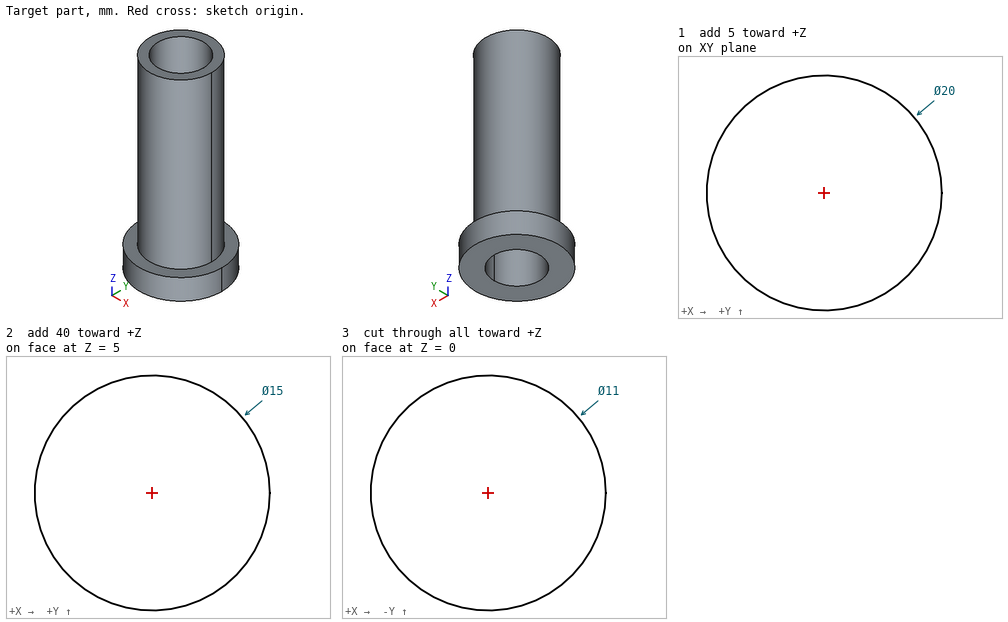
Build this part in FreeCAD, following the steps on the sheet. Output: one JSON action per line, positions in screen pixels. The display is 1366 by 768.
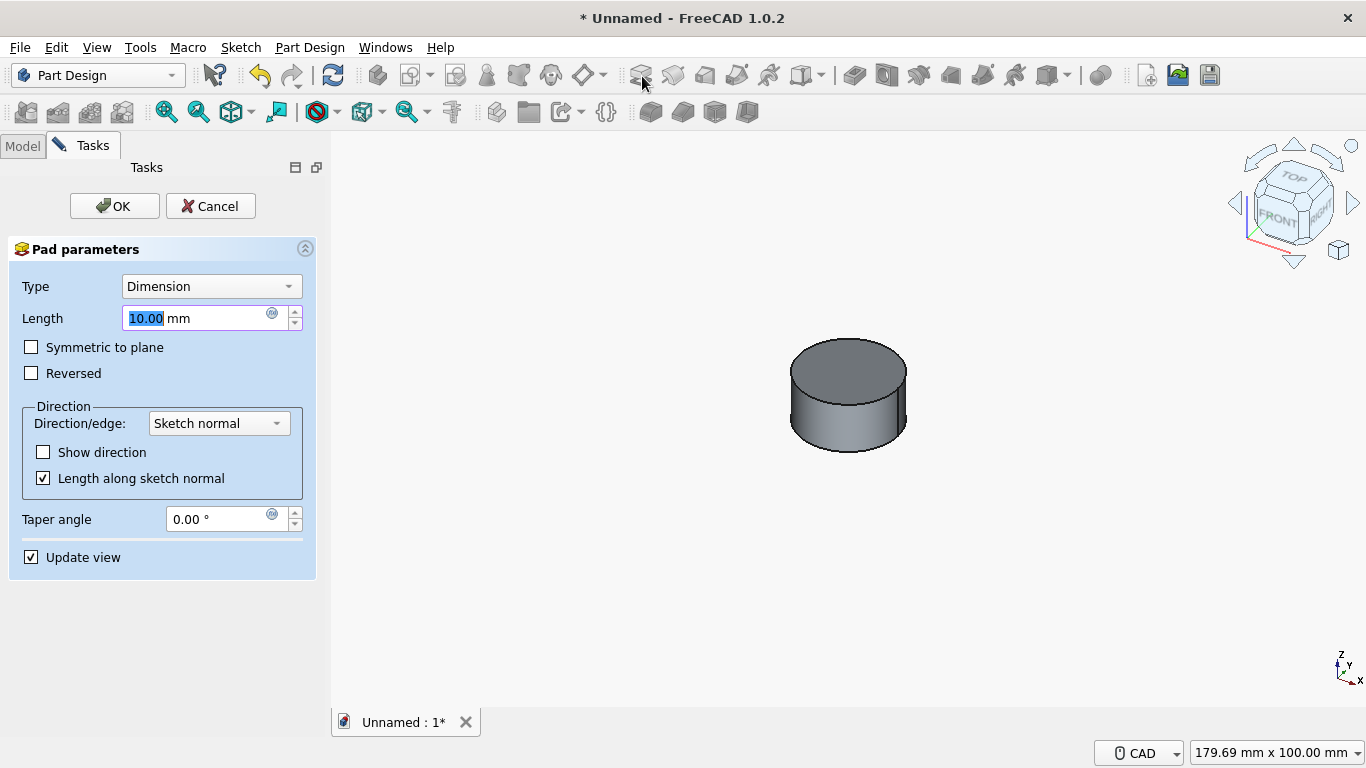
{"action": "type", "text": "5"}
{"action": "key", "text": "Tab"}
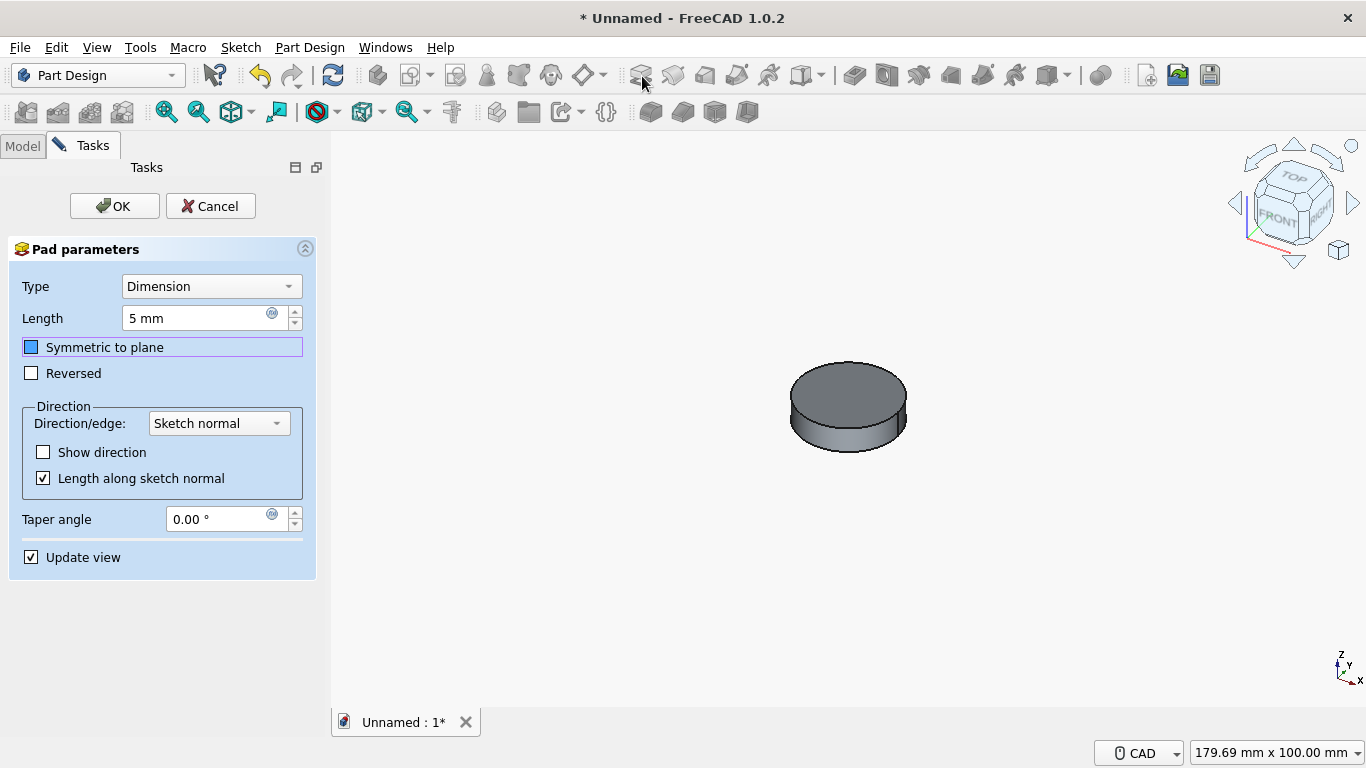
{"action": "left_click", "coordinate": [115, 206]}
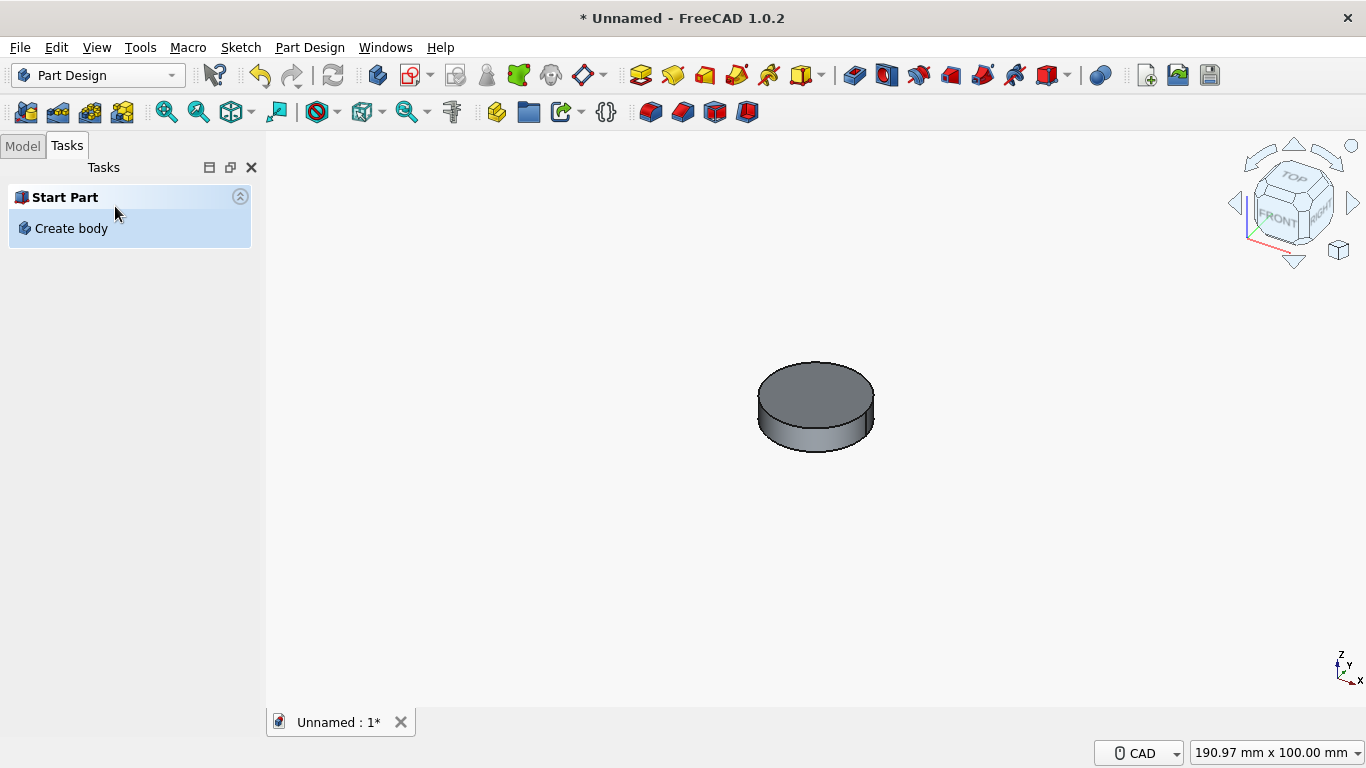
{"action": "left_click", "coordinate": [168, 112]}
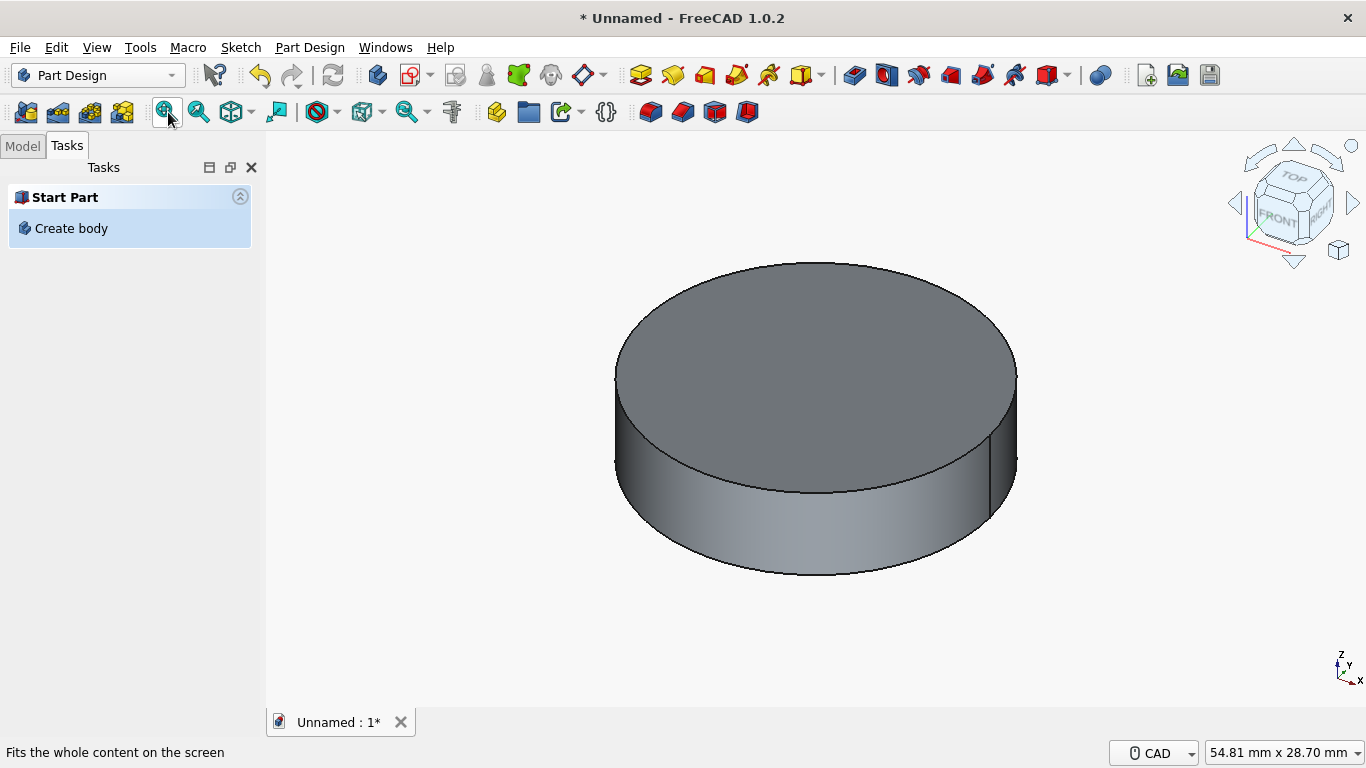
{"action": "left_click", "coordinate": [816, 377]}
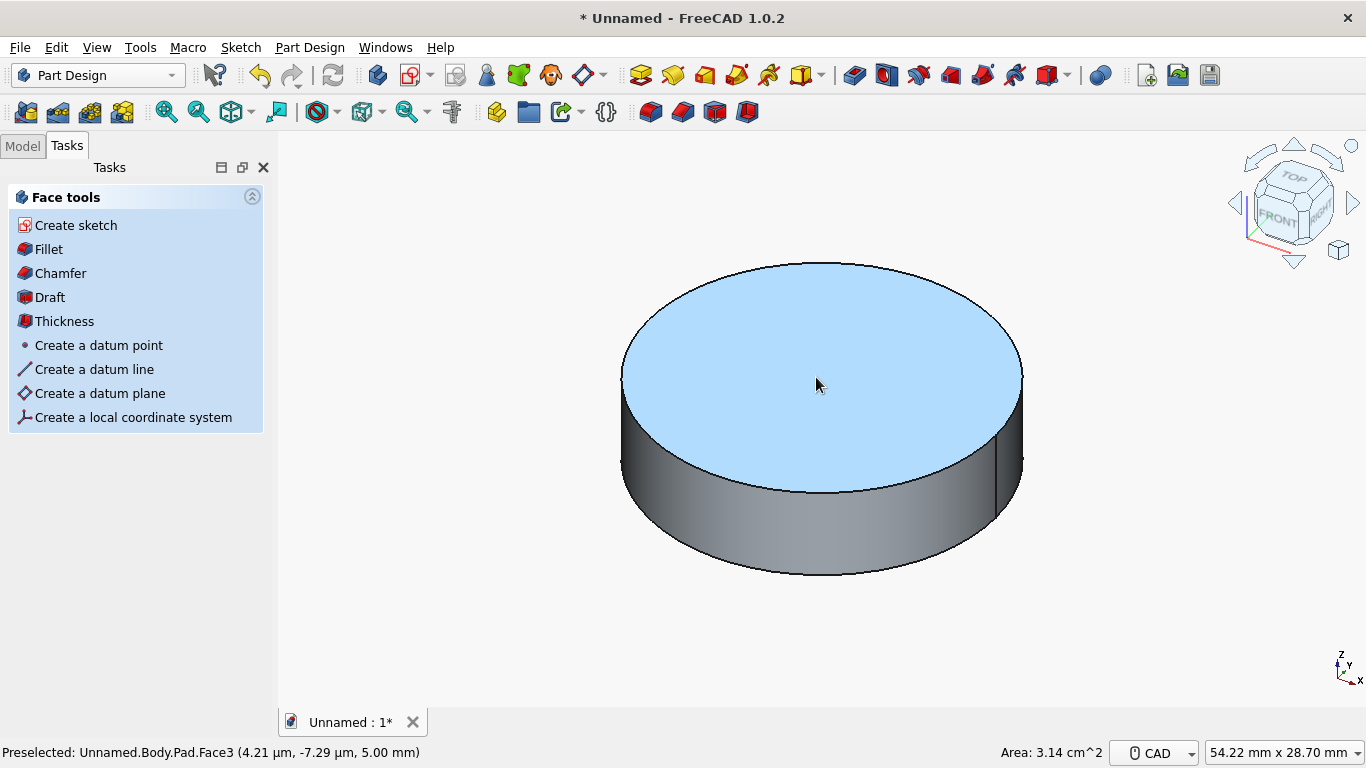
{"action": "left_click", "coordinate": [410, 76]}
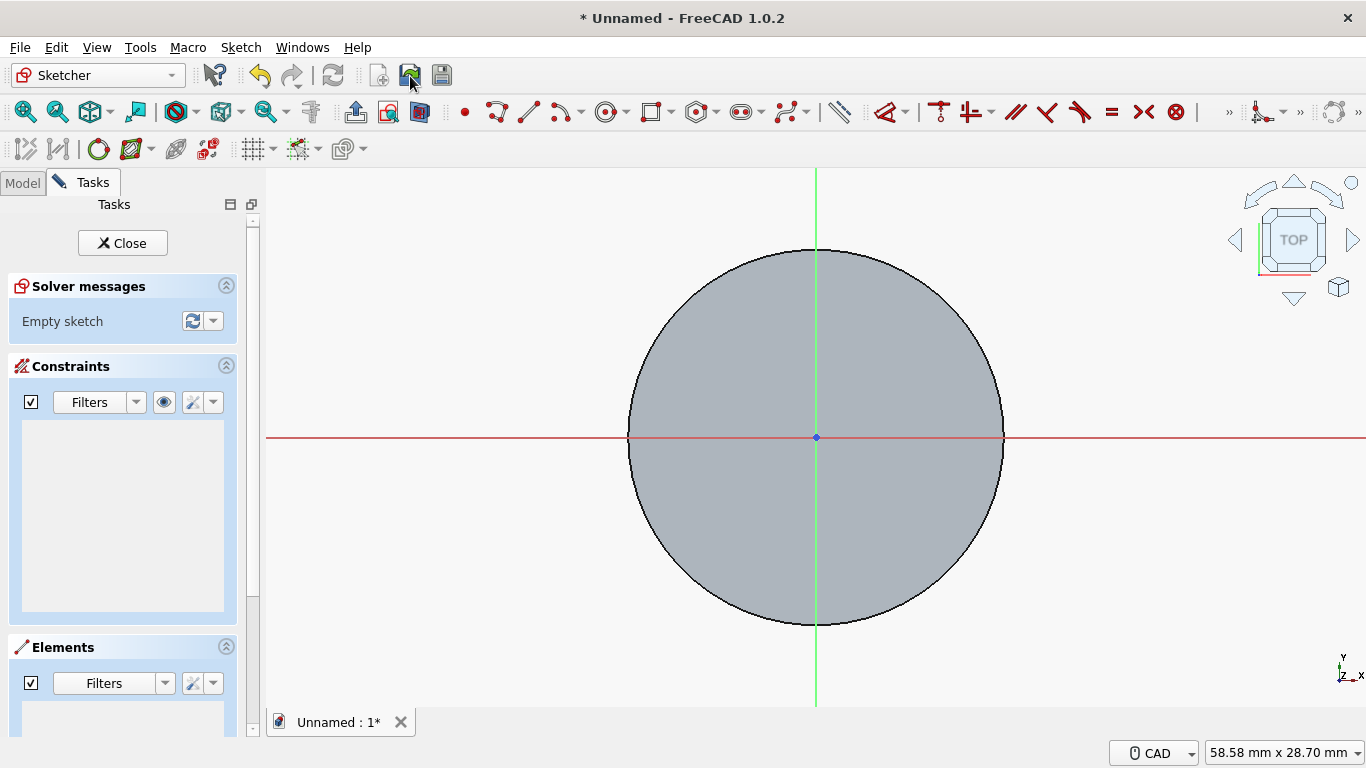
{"action": "left_click", "coordinate": [606, 112]}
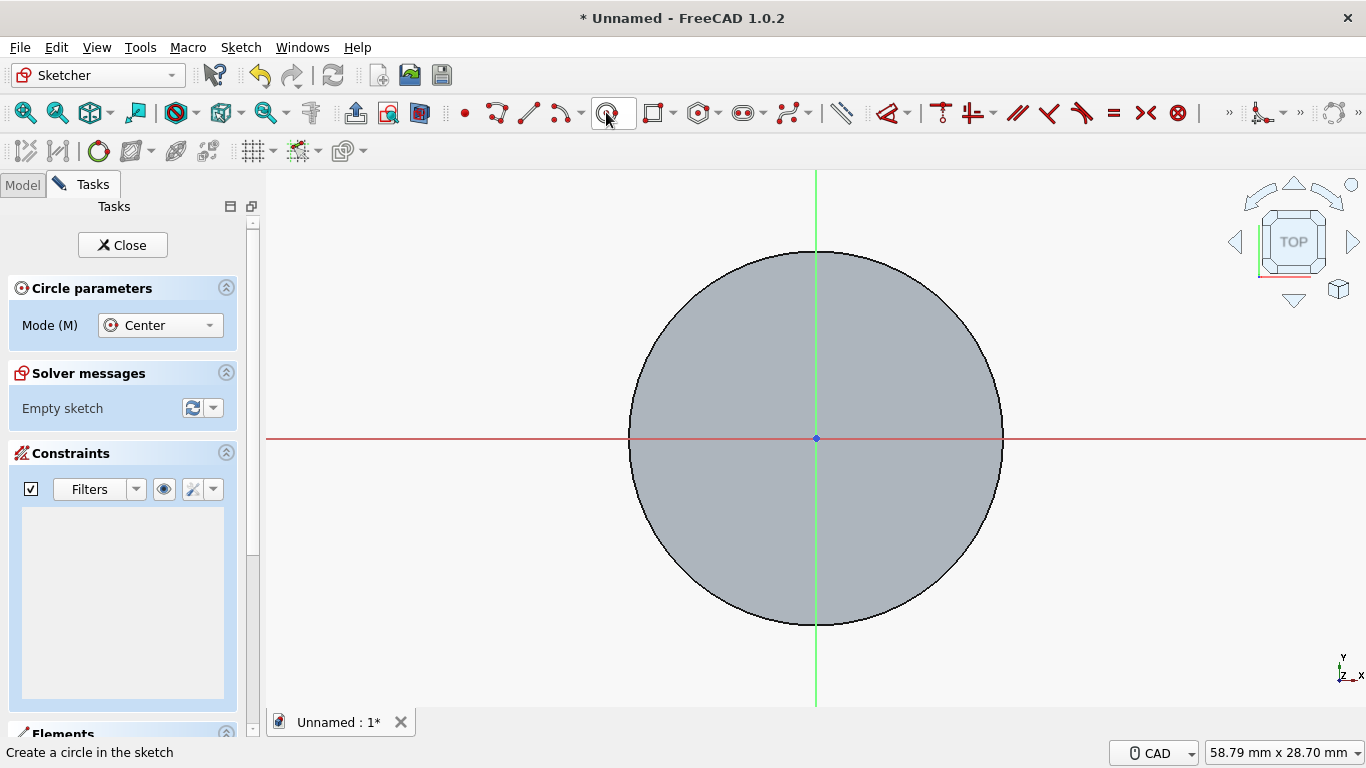
{"action": "left_click", "coordinate": [816, 438]}
{"action": "mouse_move", "coordinate": [915, 339]}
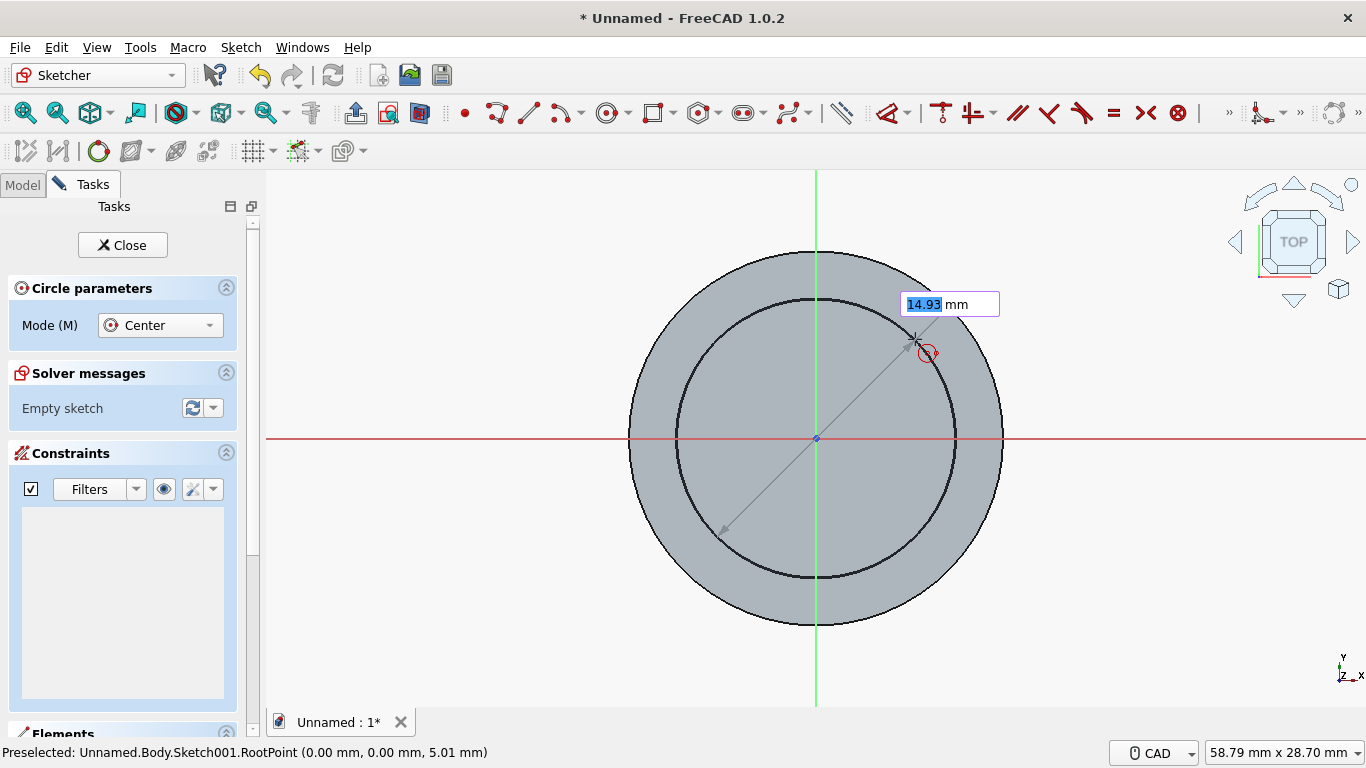
{"action": "type", "text": "15"}
{"action": "key", "text": "Return"}
{"action": "key", "text": "Escape"}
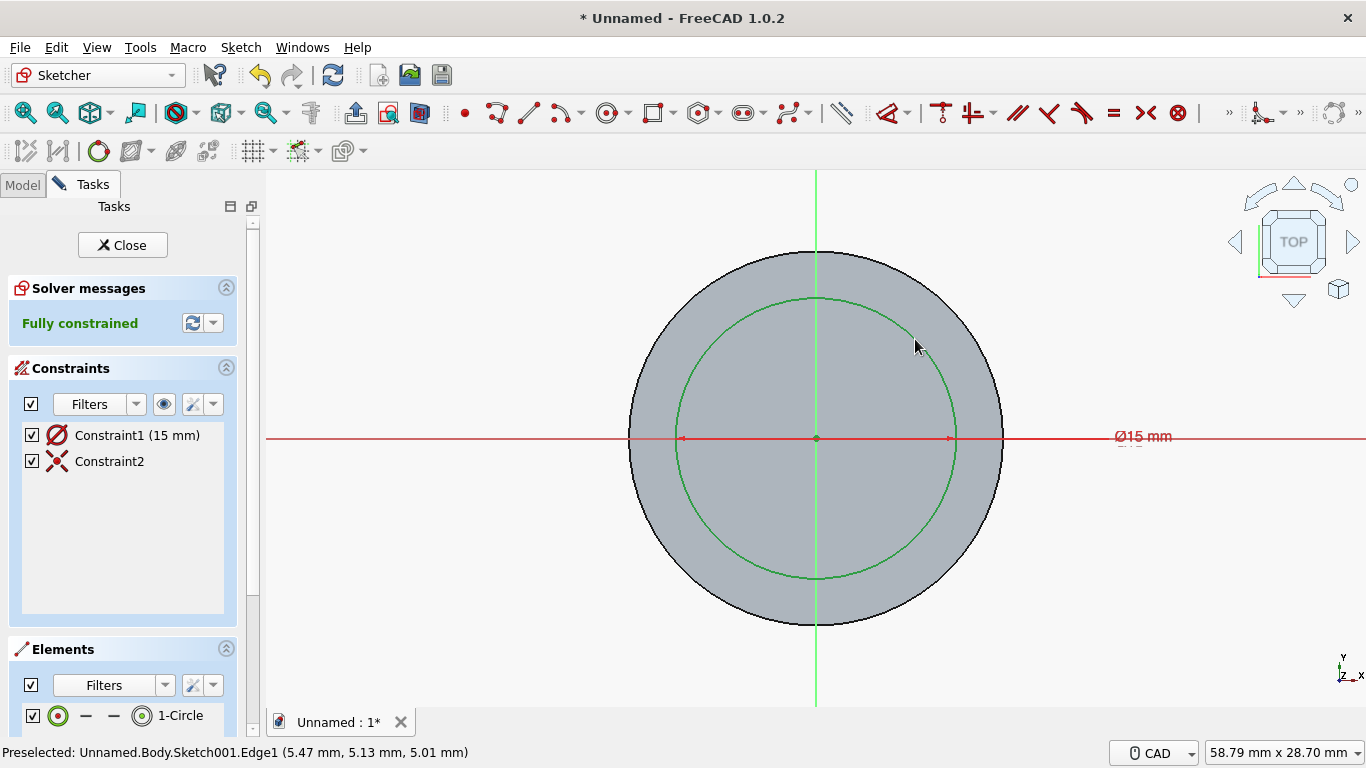
{"action": "left_click", "coordinate": [123, 245]}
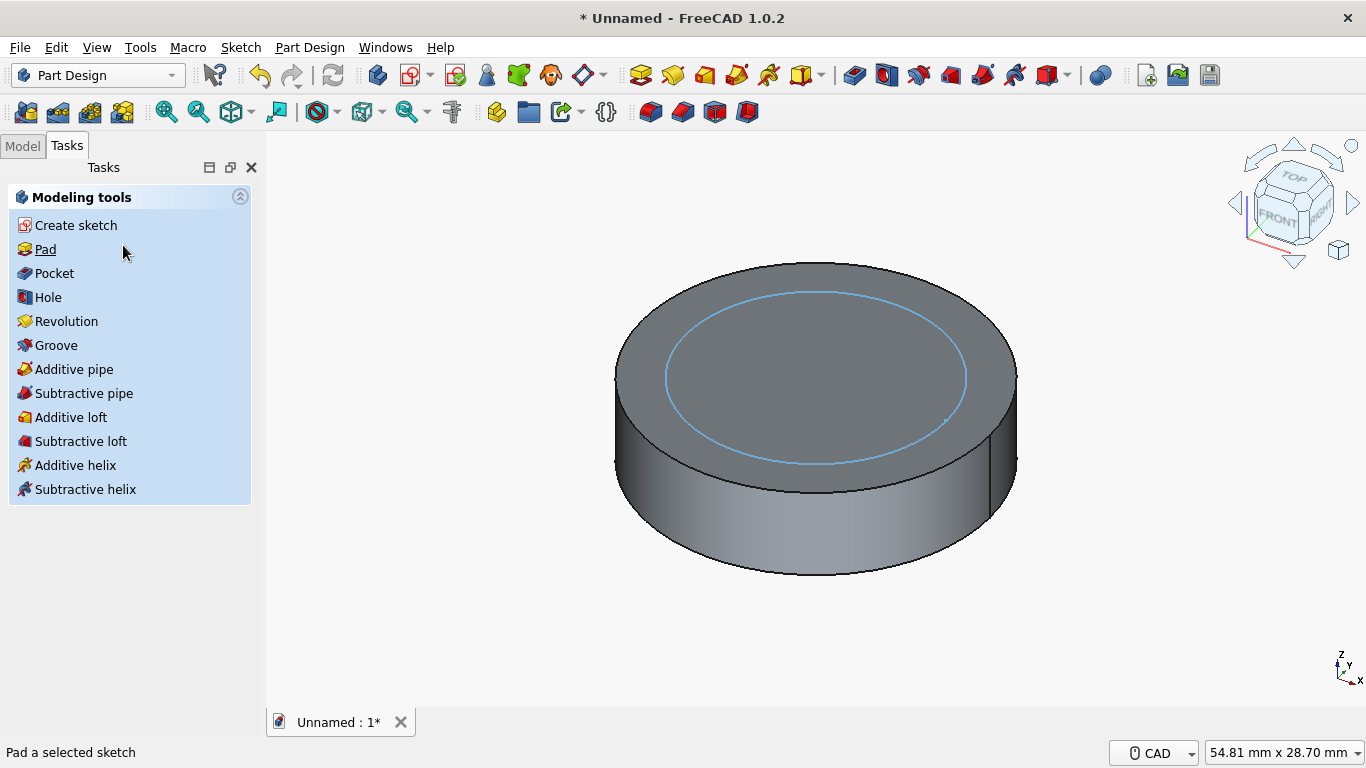
{"action": "left_click", "coordinate": [642, 76]}